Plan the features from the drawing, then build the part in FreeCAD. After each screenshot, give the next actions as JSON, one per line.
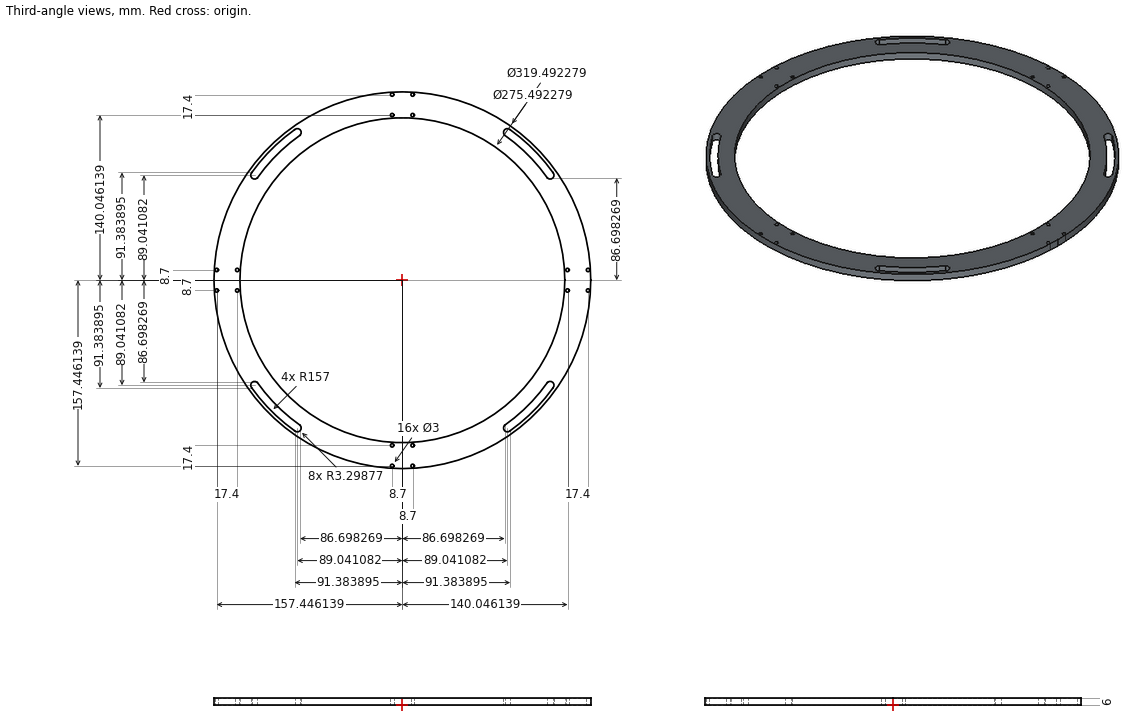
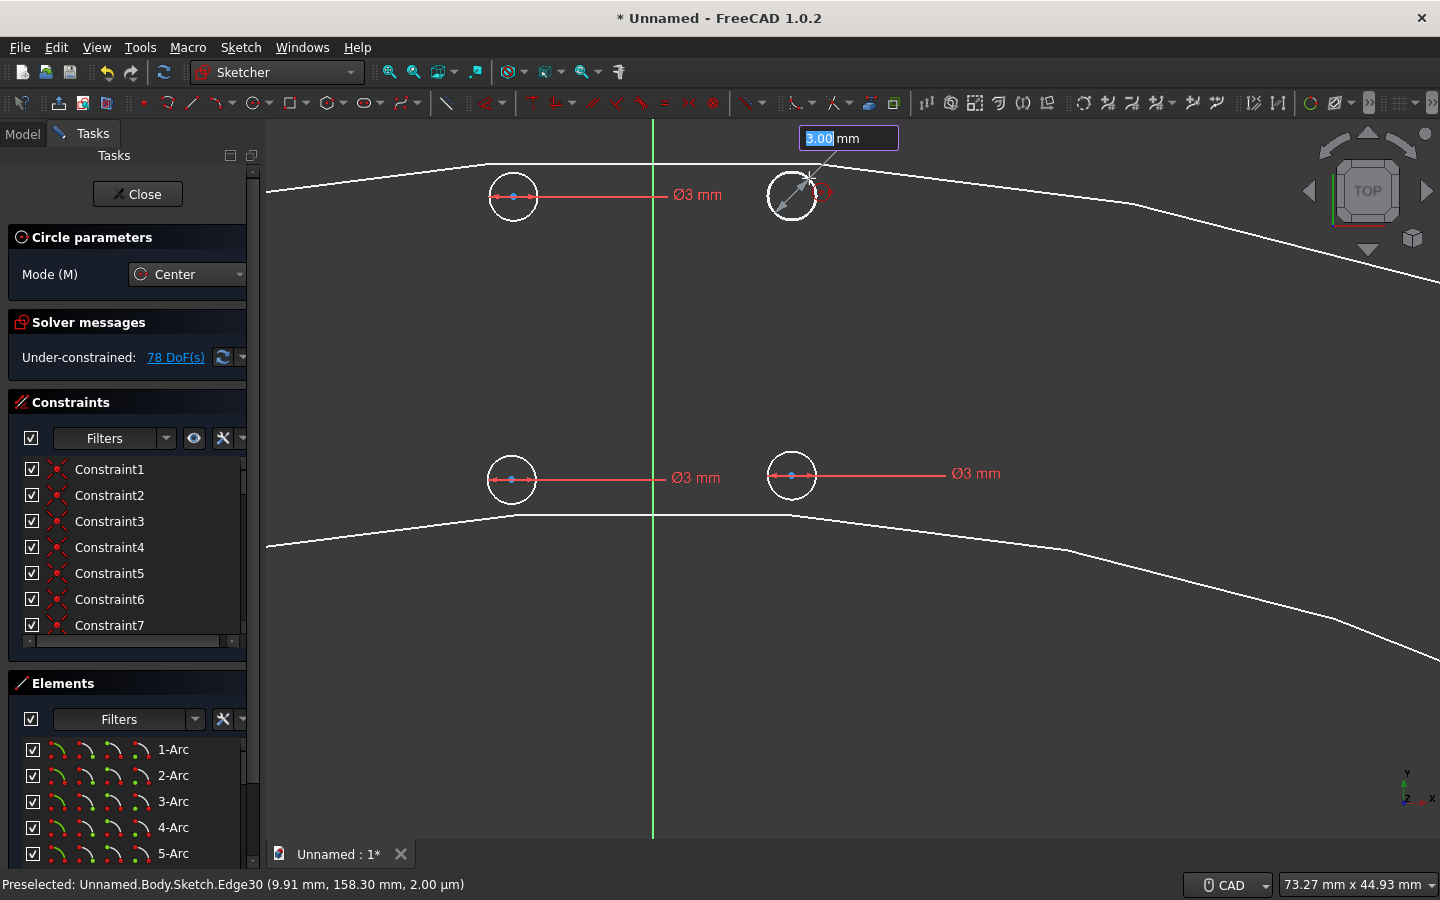
{"action": "type", "text": "3"}
{"action": "key", "text": "Return"}
{"action": "key", "text": "Escape"}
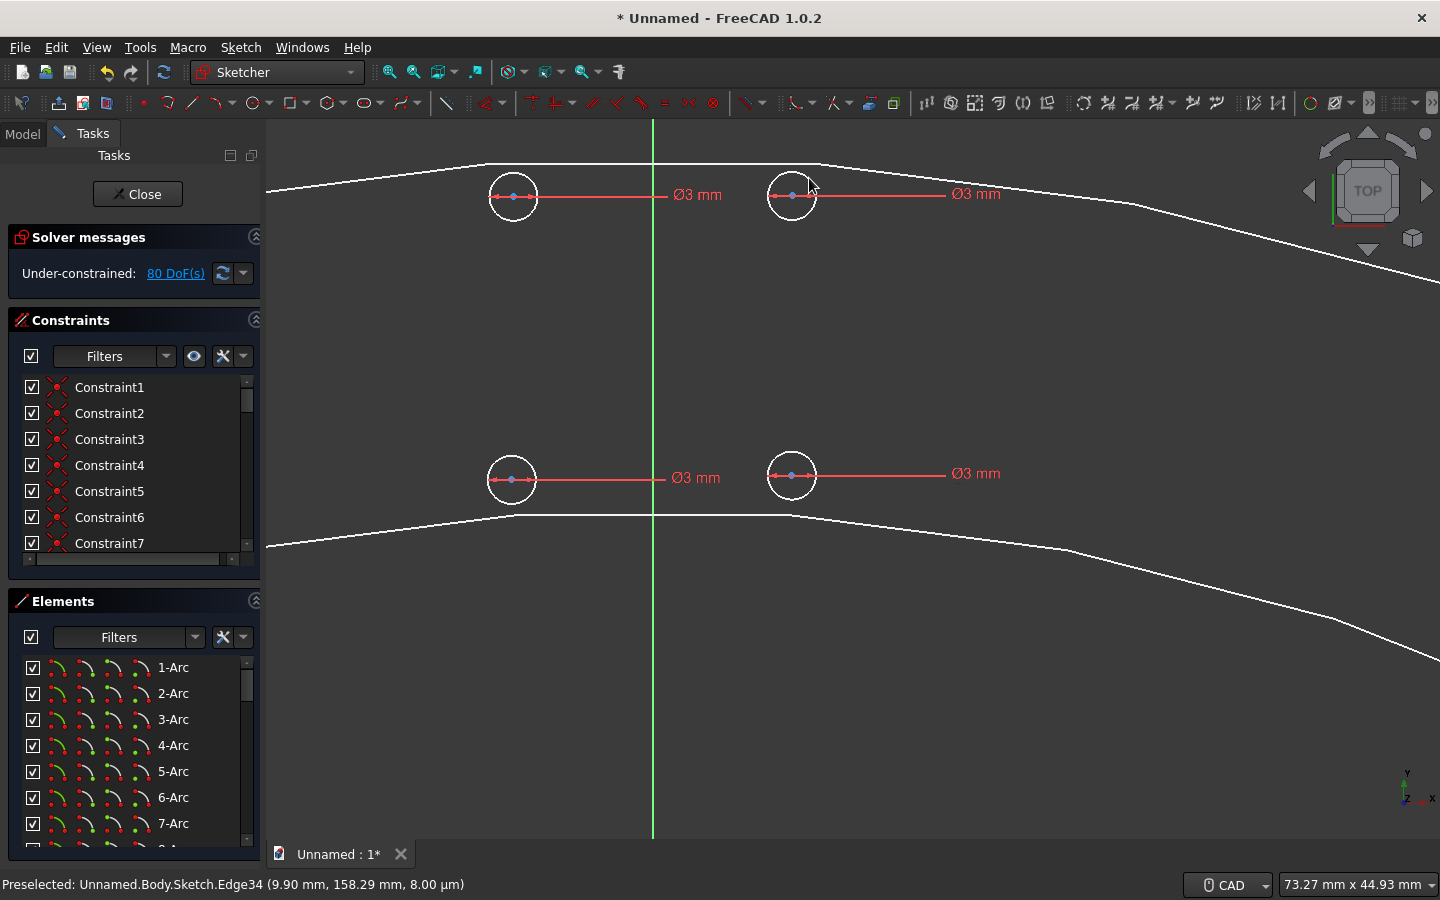
{"action": "scroll", "coordinate": [798, 256], "scroll_direction": "down", "scroll_amount": 12}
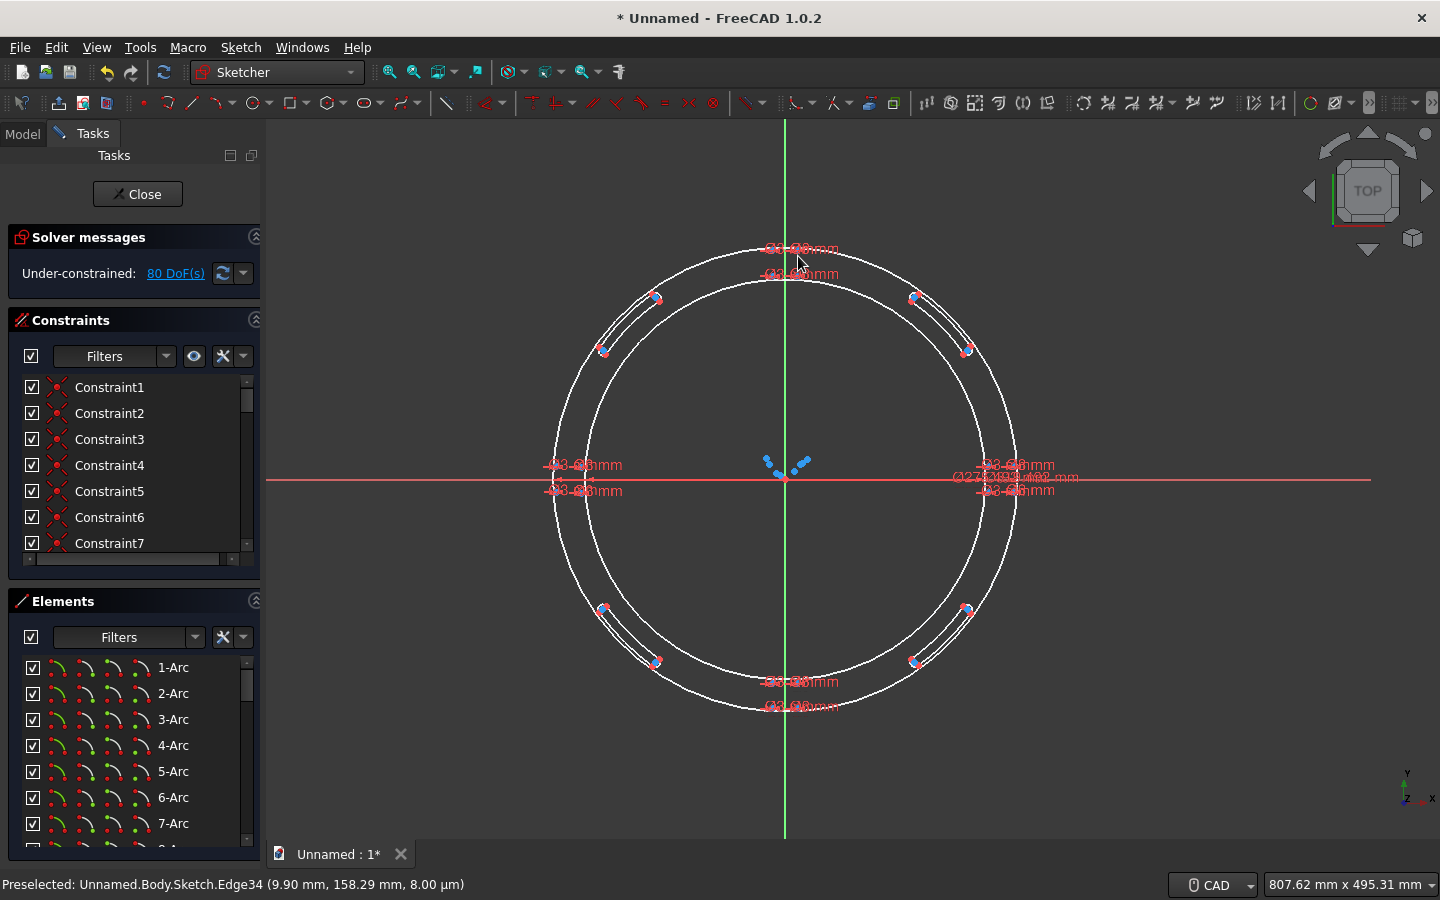
{"action": "scroll", "coordinate": [792, 247], "scroll_direction": "up", "scroll_amount": 6}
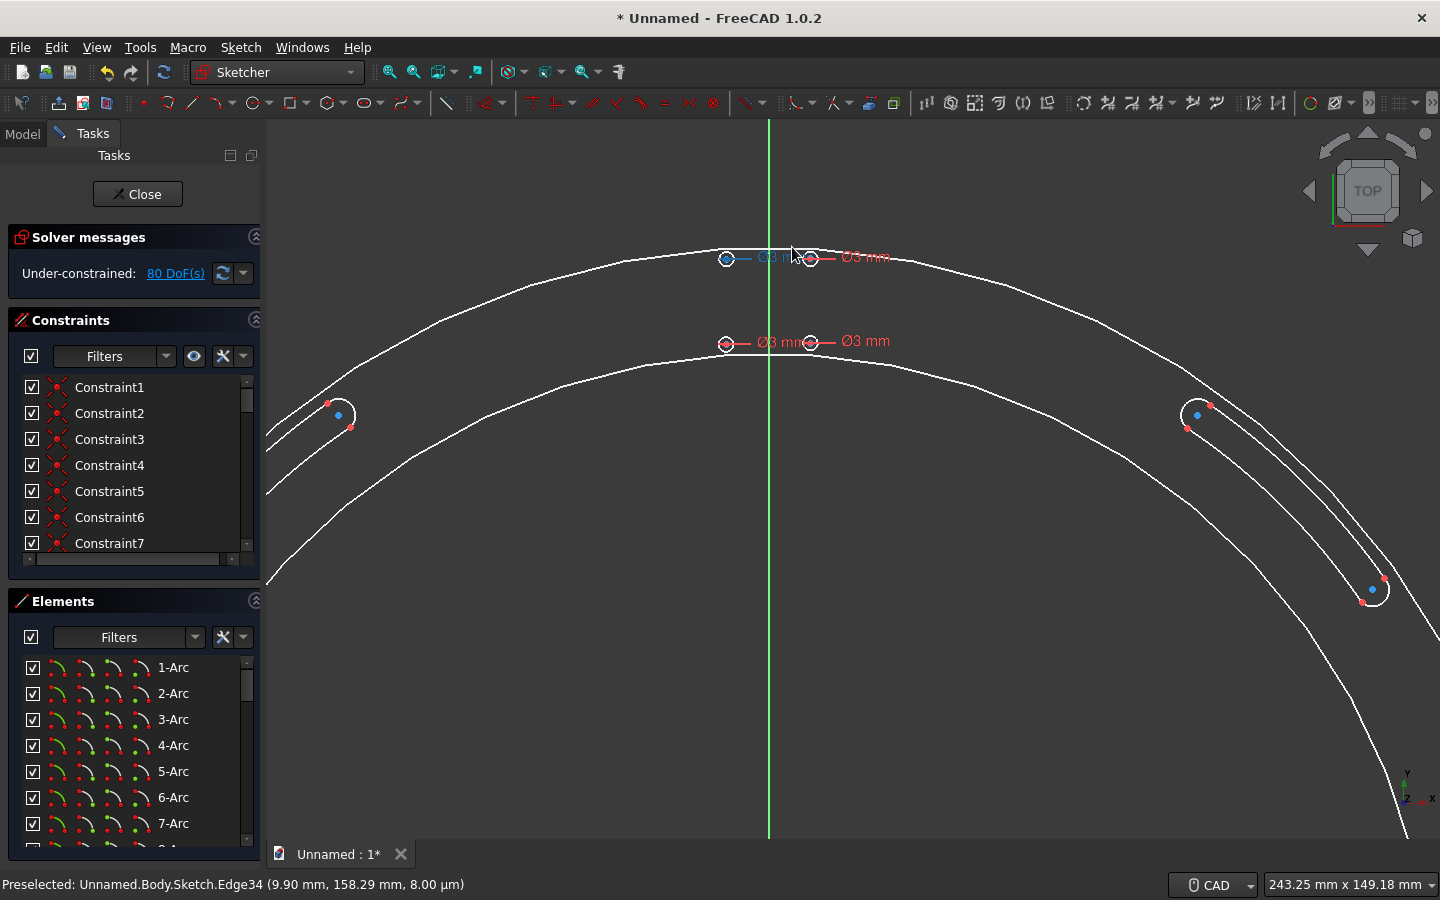
{"action": "left_click", "coordinate": [790, 248]}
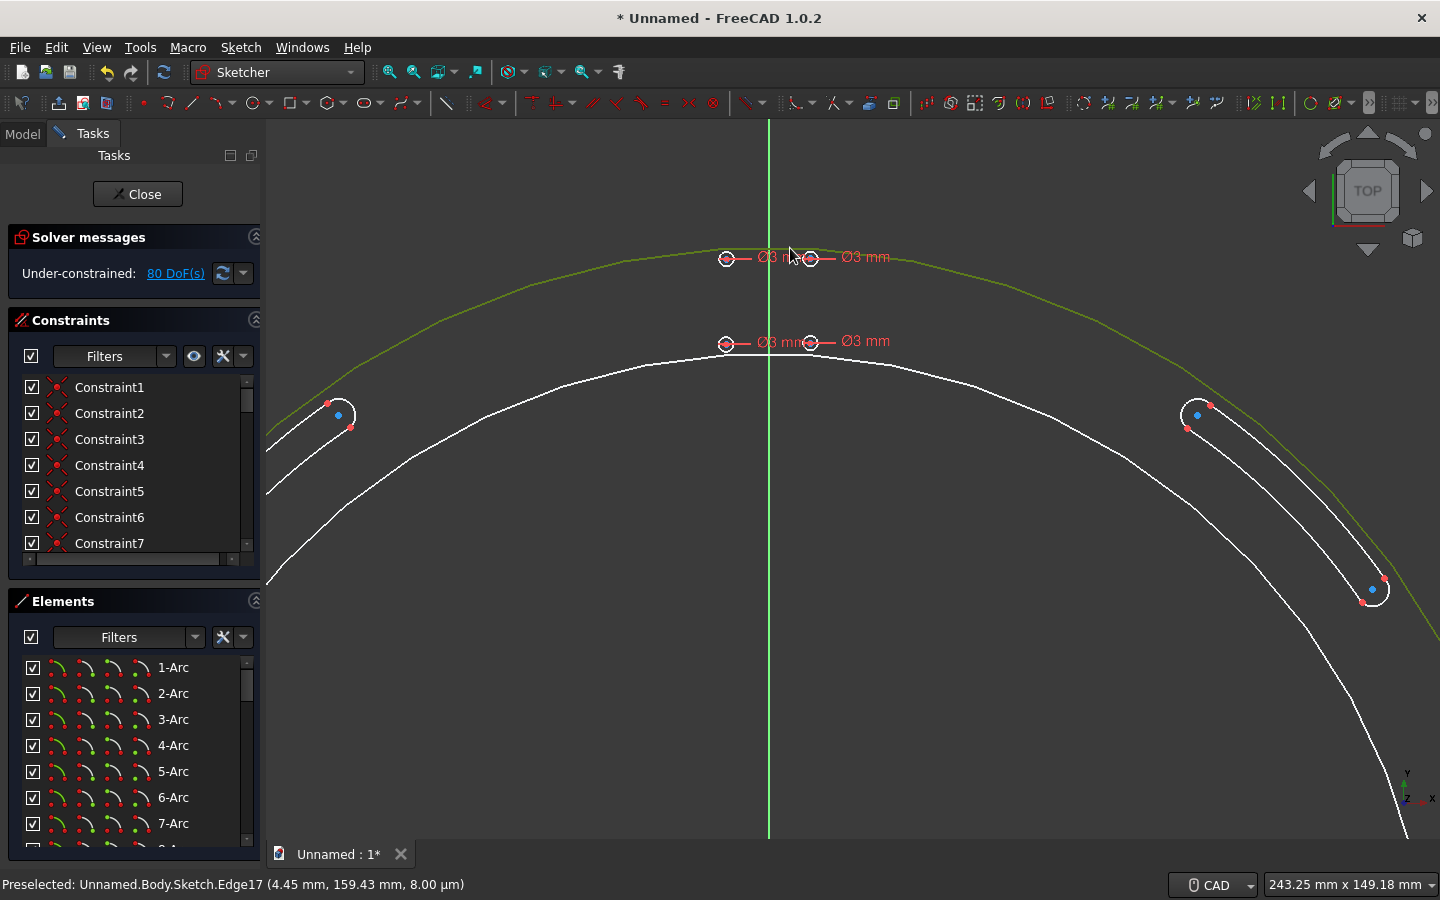
{"action": "scroll", "coordinate": [791, 246], "scroll_direction": "down", "scroll_amount": 6}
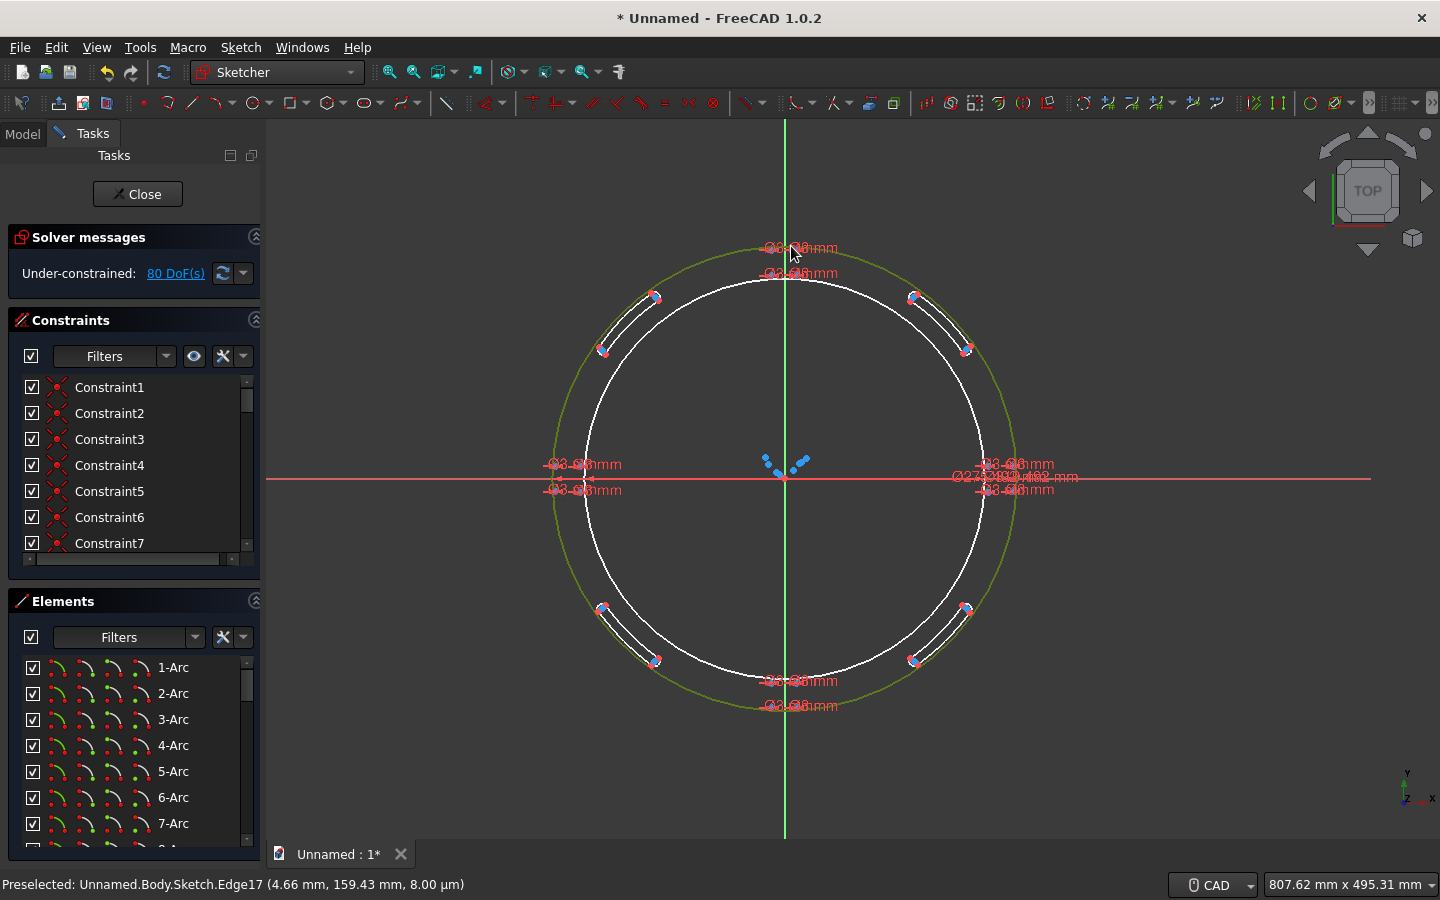
{"action": "scroll", "coordinate": [613, 630], "scroll_direction": "up", "scroll_amount": 7}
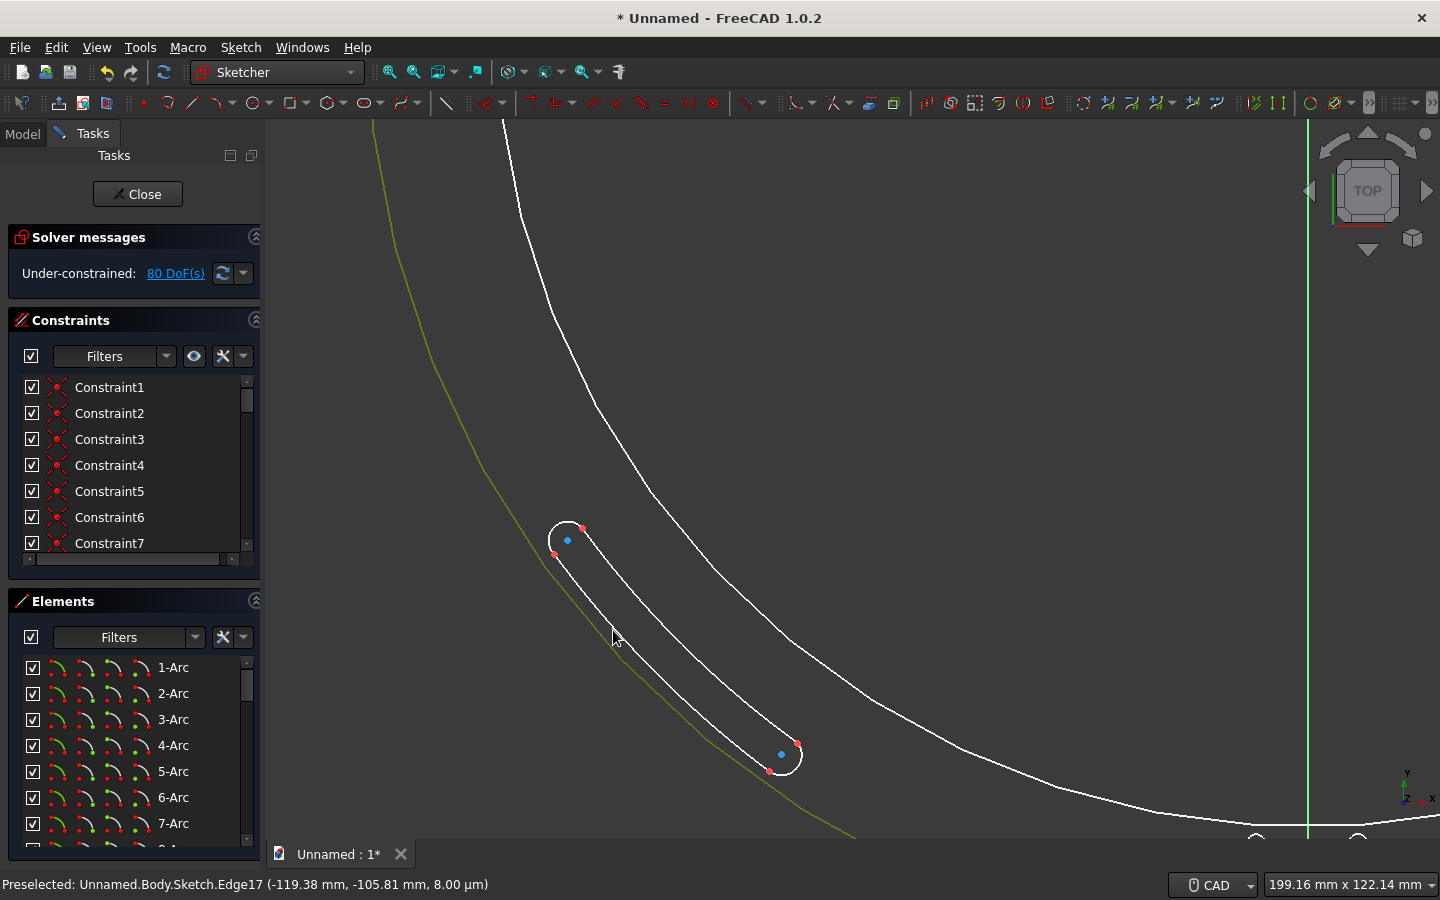
{"action": "left_click", "coordinate": [612, 626]}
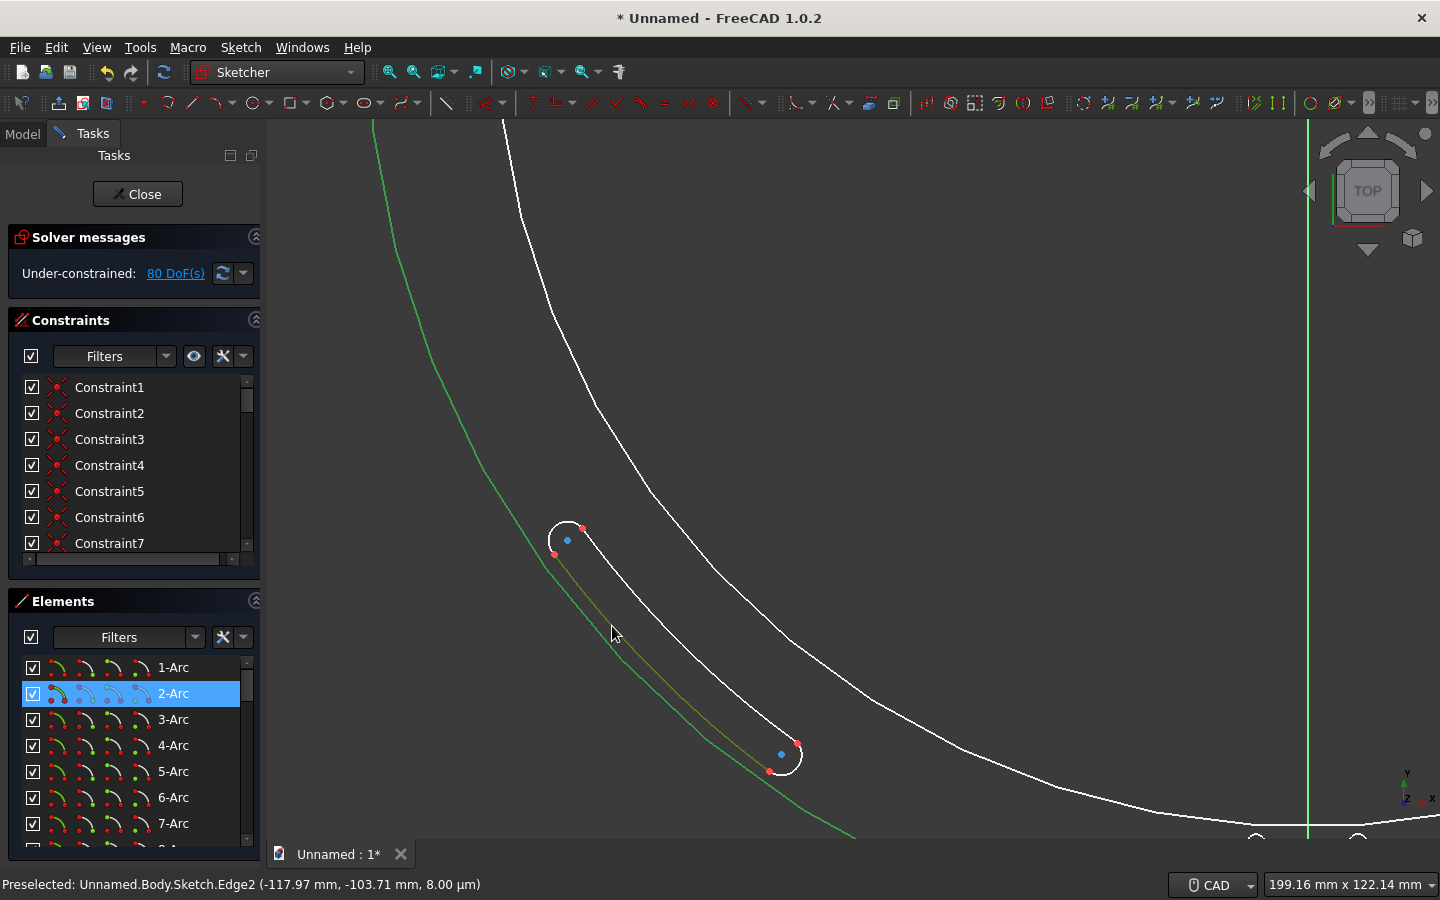
{"action": "key", "text": "c"}